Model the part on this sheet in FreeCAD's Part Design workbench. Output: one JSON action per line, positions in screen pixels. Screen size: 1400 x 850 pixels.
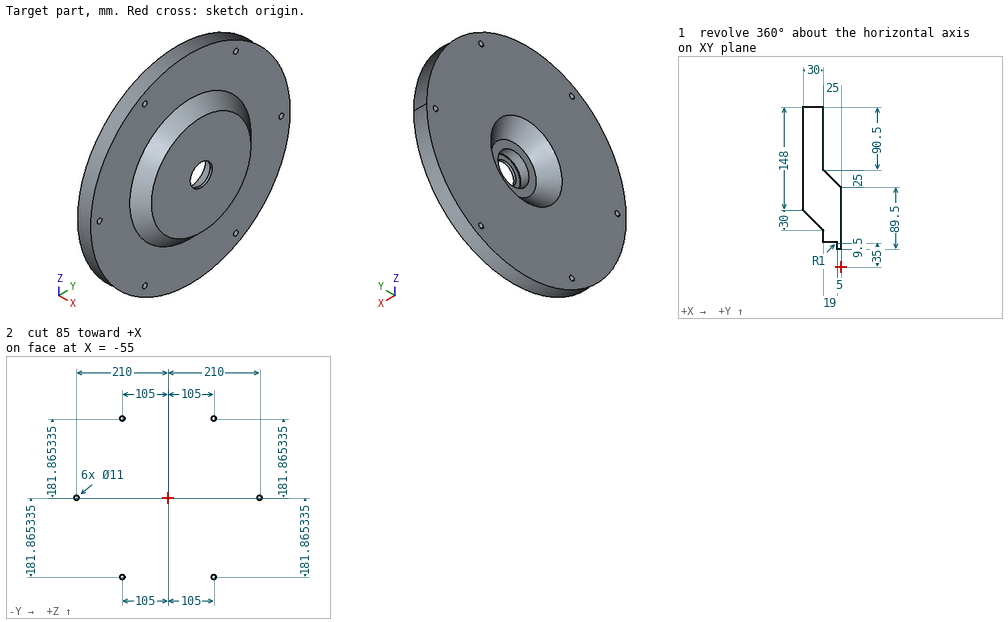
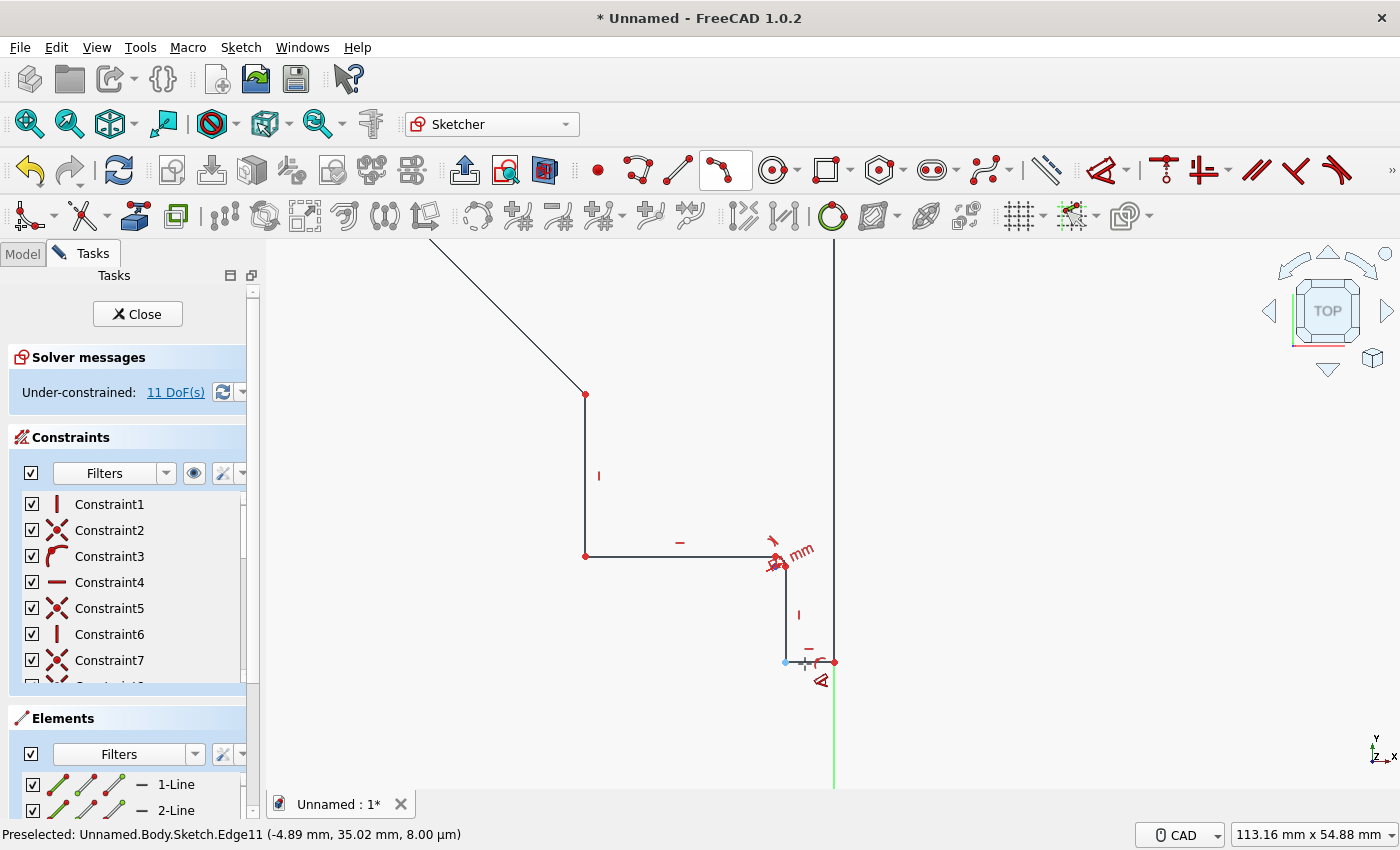
{"action": "left_click", "coordinate": [800, 662]}
{"action": "left_click", "coordinate": [810, 696]}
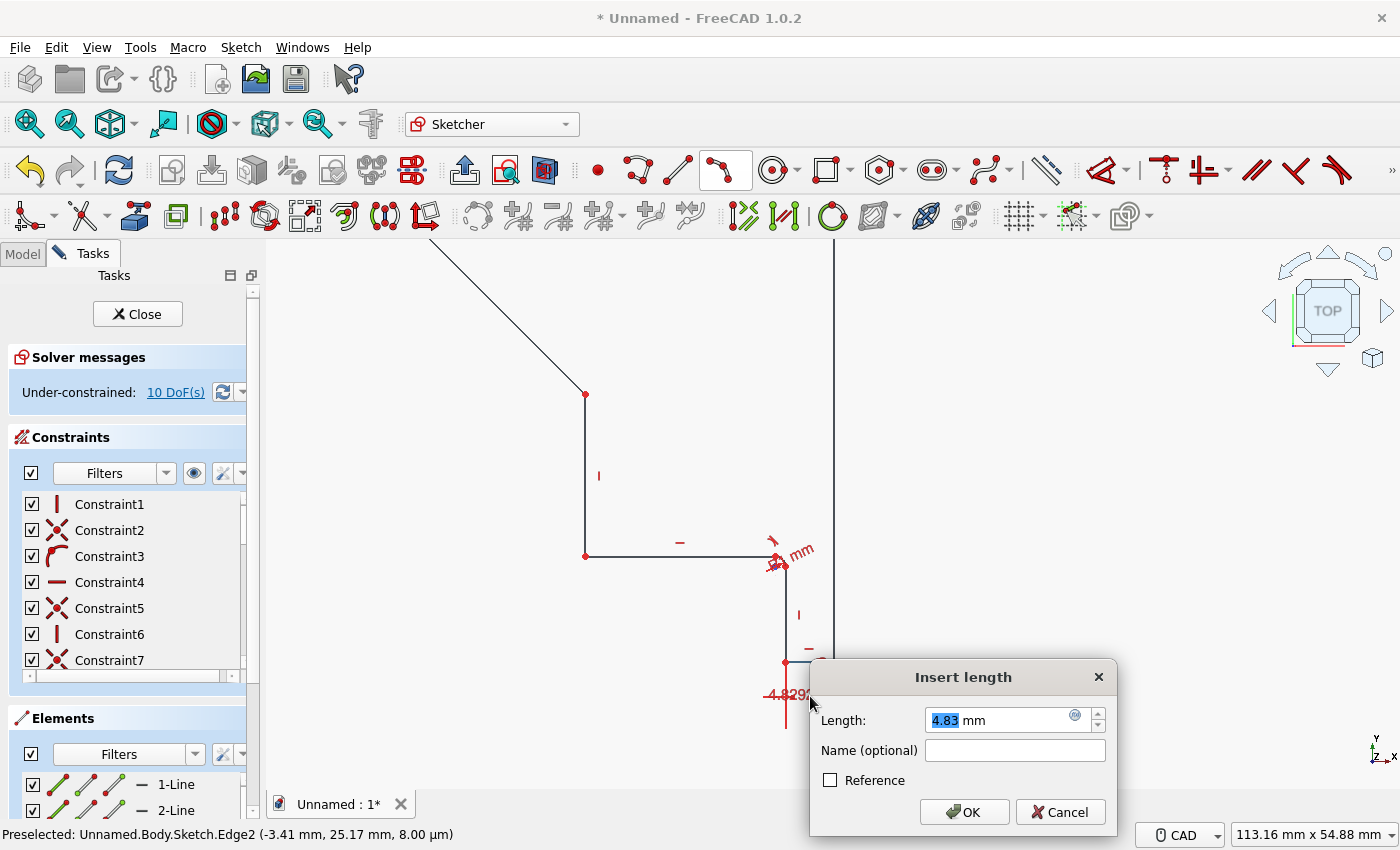
{"action": "type", "text": "5"}
{"action": "key", "text": "Return"}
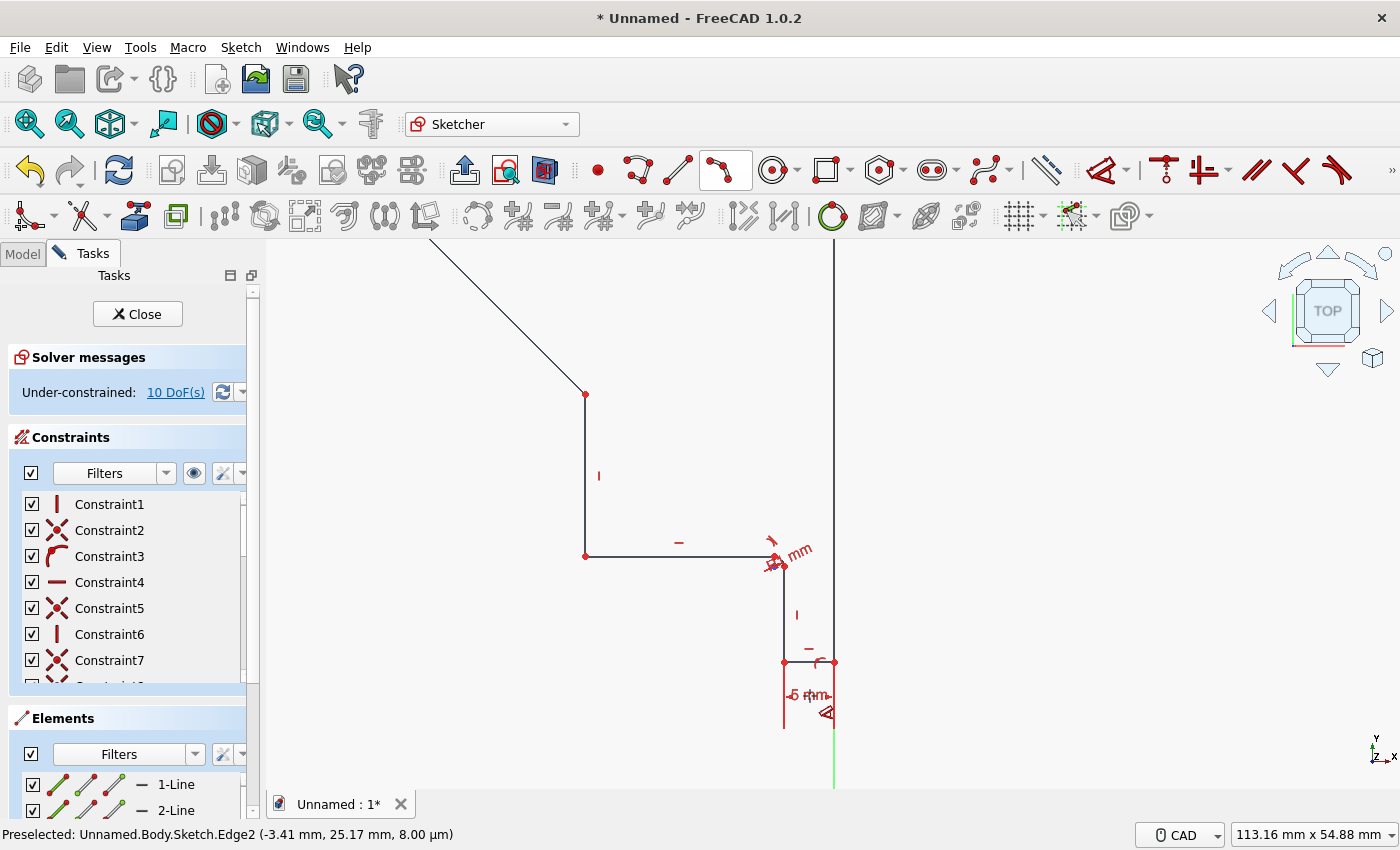
{"action": "scroll", "coordinate": [805, 663], "scroll_direction": "down", "scroll_amount": 9}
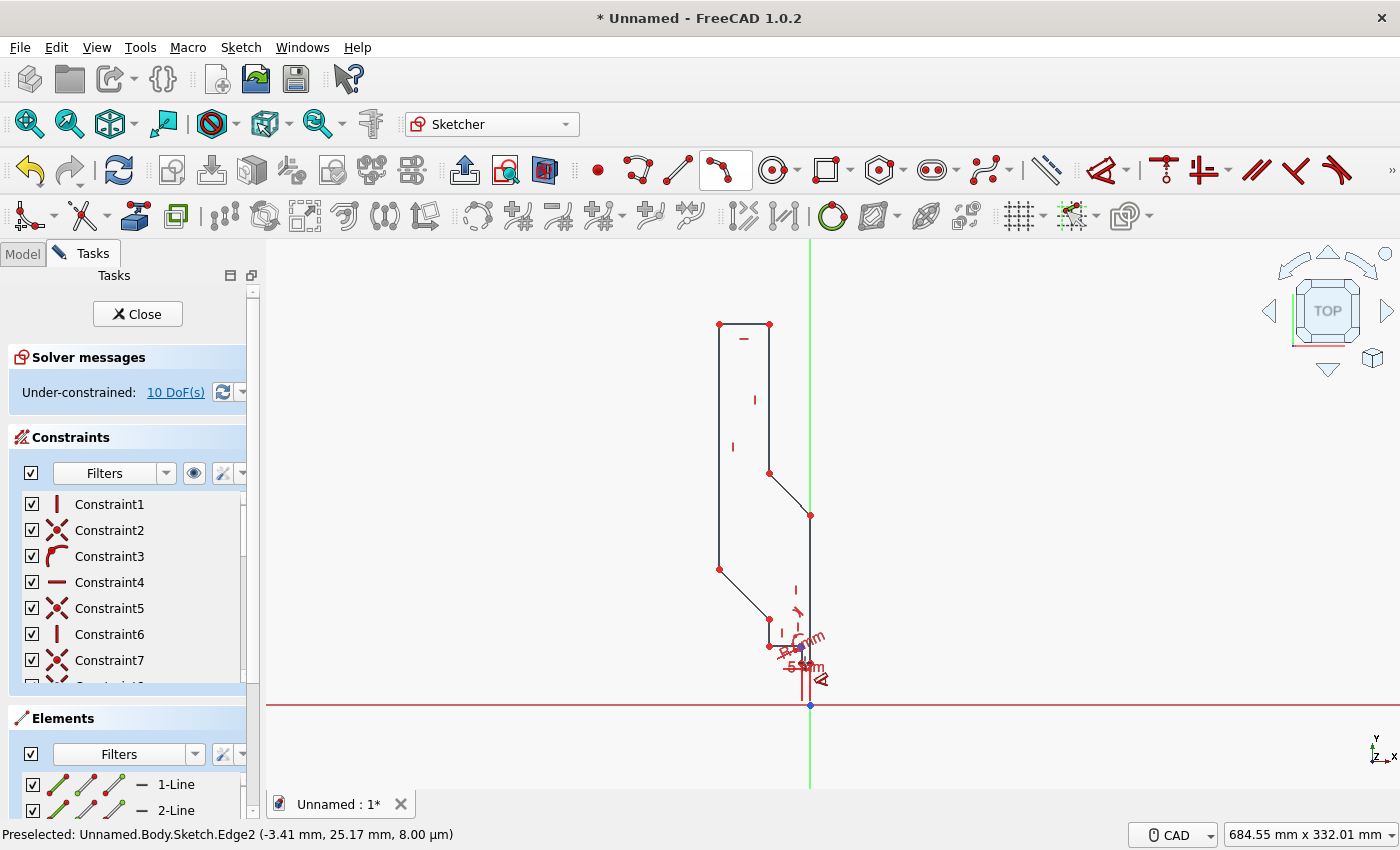
{"action": "left_click", "coordinate": [754, 324]}
{"action": "left_click", "coordinate": [744, 290]}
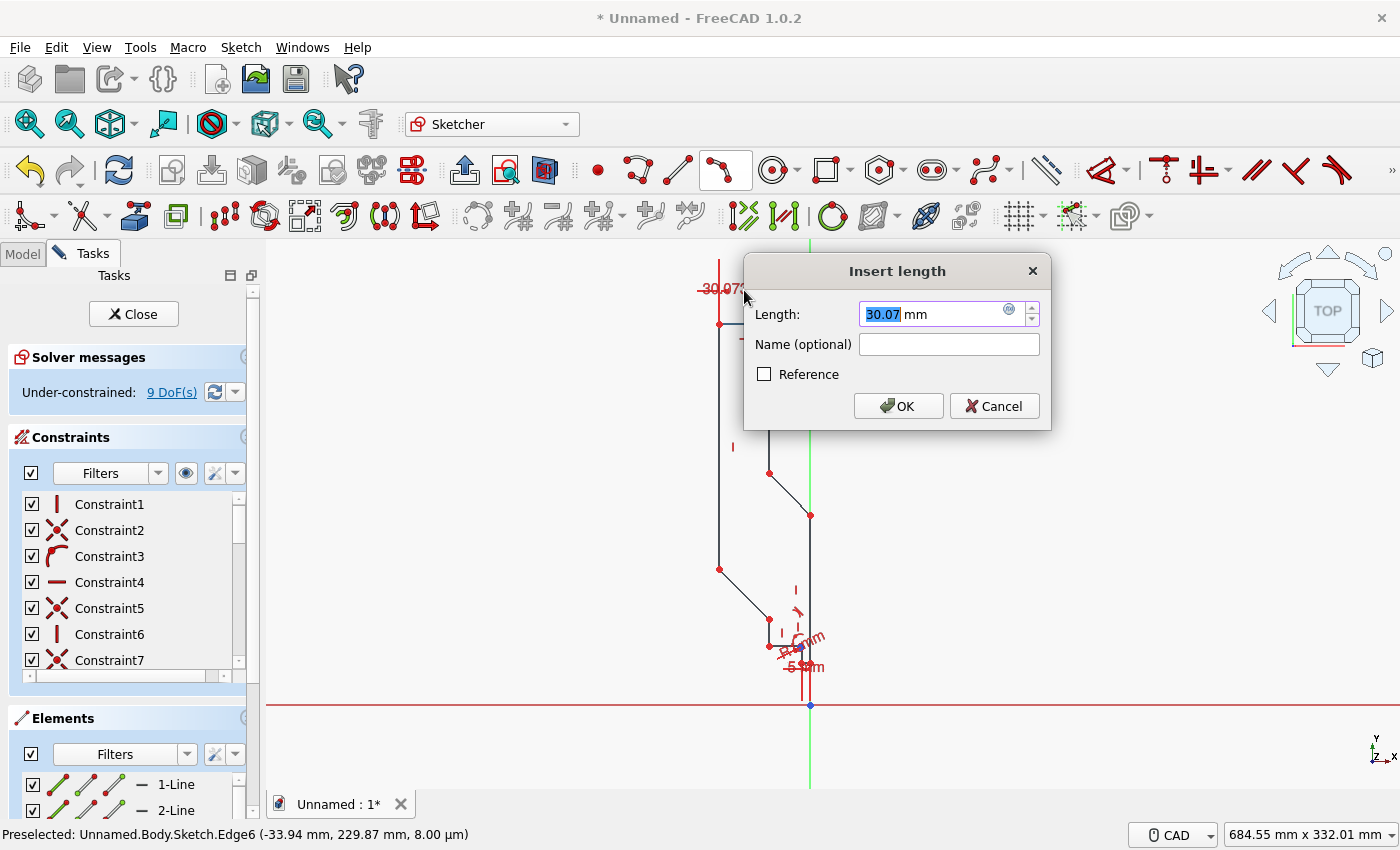
{"action": "type", "text": "30"}
{"action": "key", "text": "Return"}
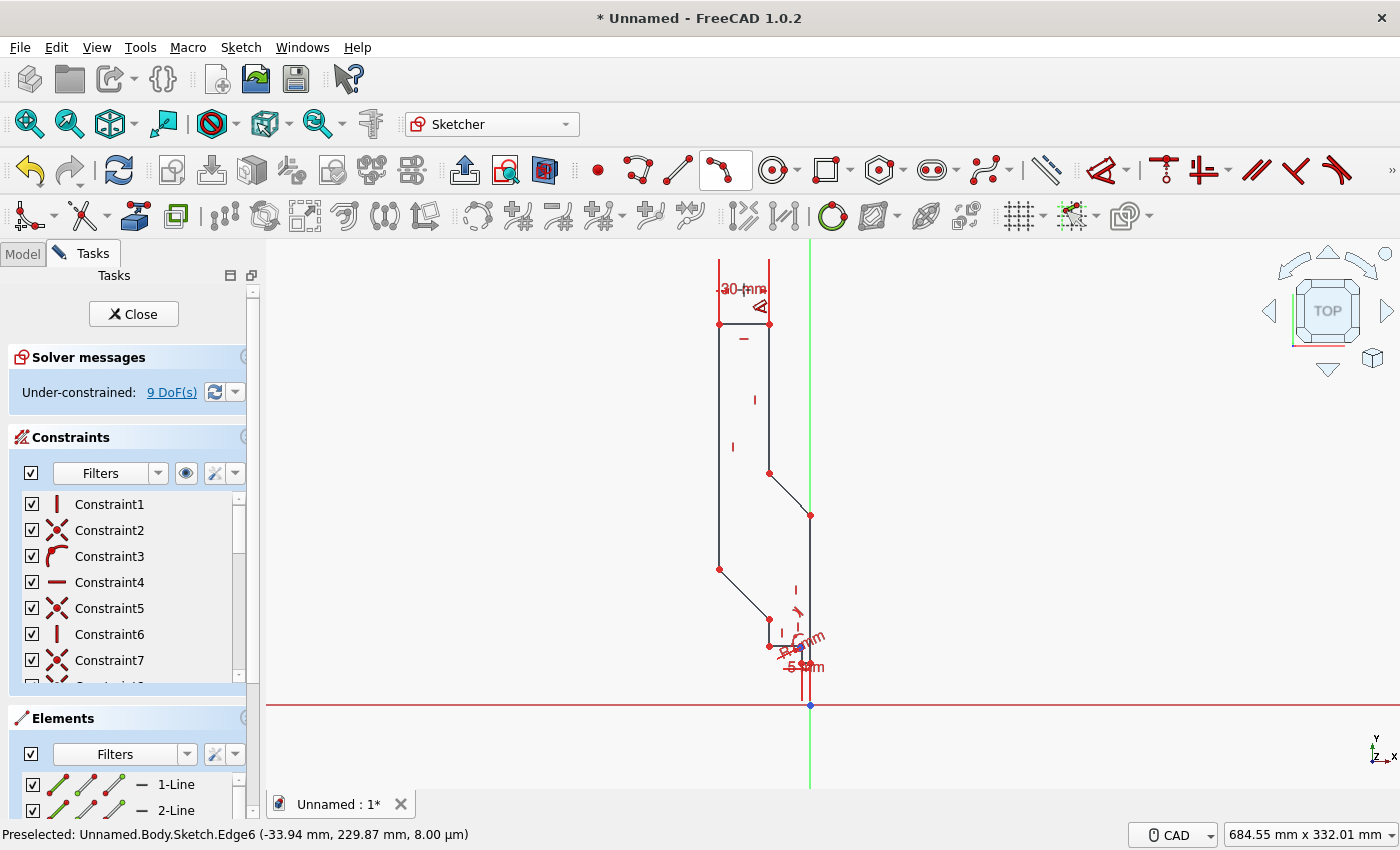
{"action": "scroll", "coordinate": [778, 646], "scroll_direction": "up", "scroll_amount": 2}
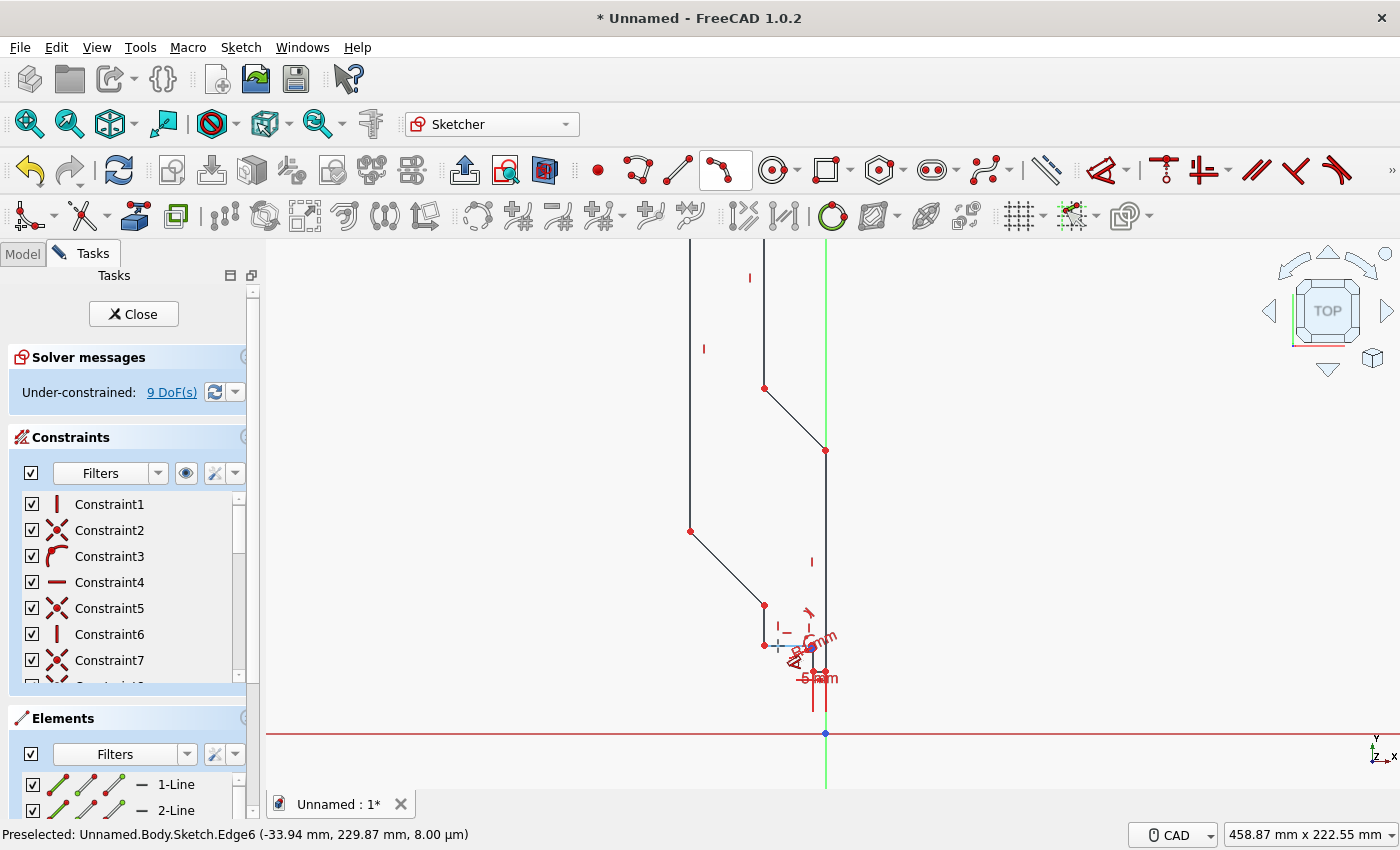
{"action": "left_click", "coordinate": [778, 646]}
{"action": "left_click", "coordinate": [788, 612]}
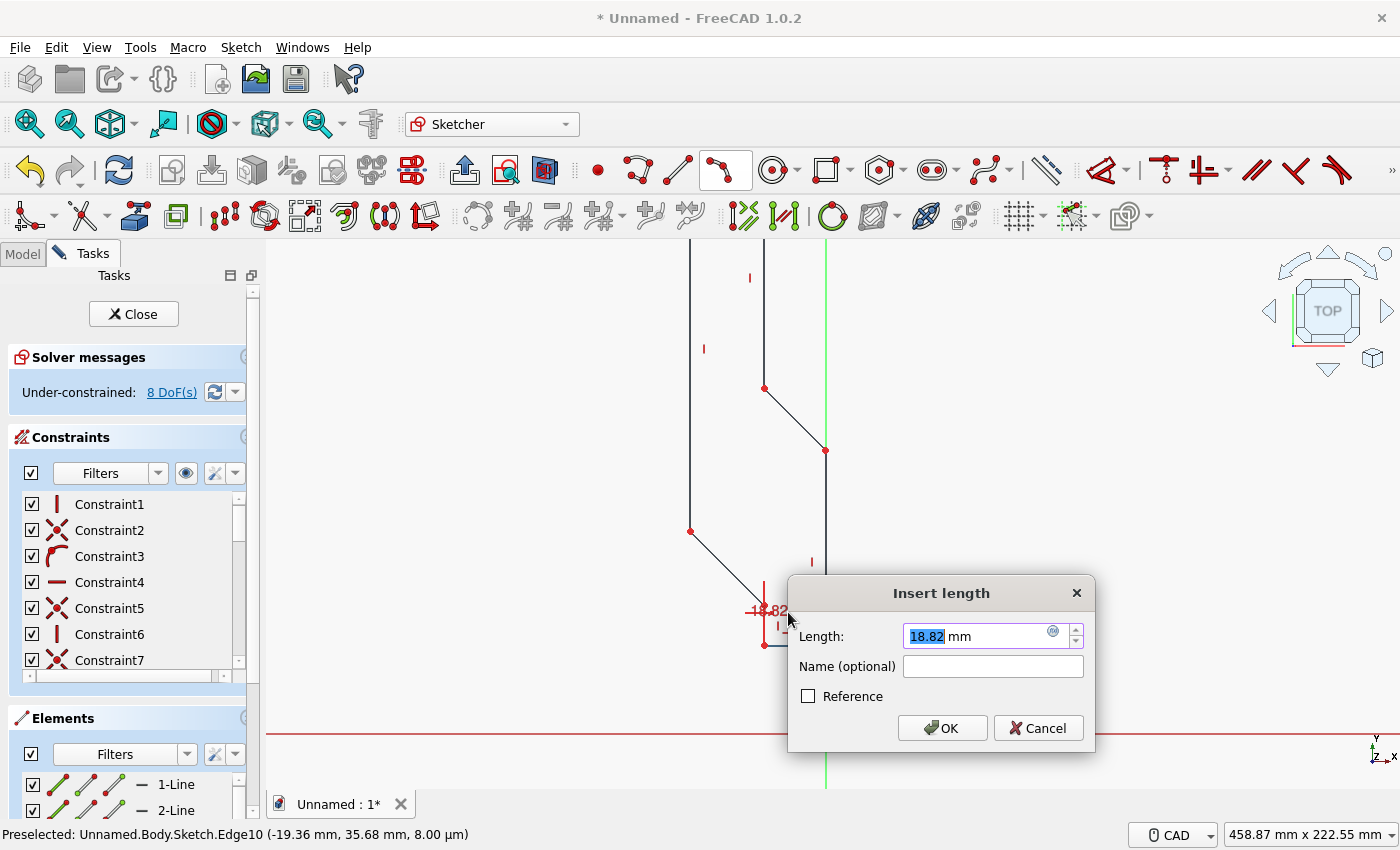
{"action": "type", "text": "19"}
{"action": "key", "text": "Return"}